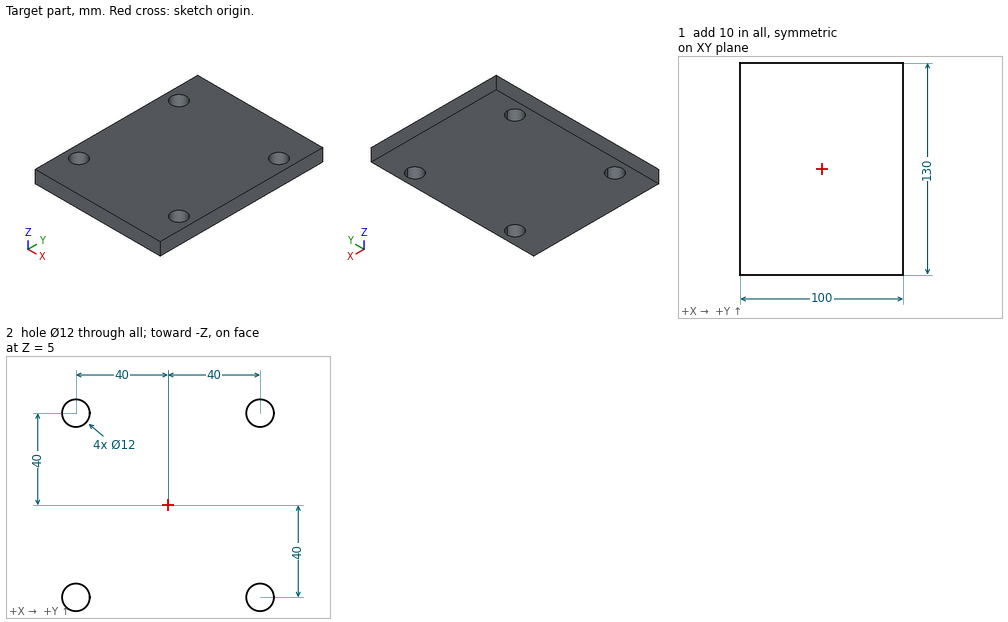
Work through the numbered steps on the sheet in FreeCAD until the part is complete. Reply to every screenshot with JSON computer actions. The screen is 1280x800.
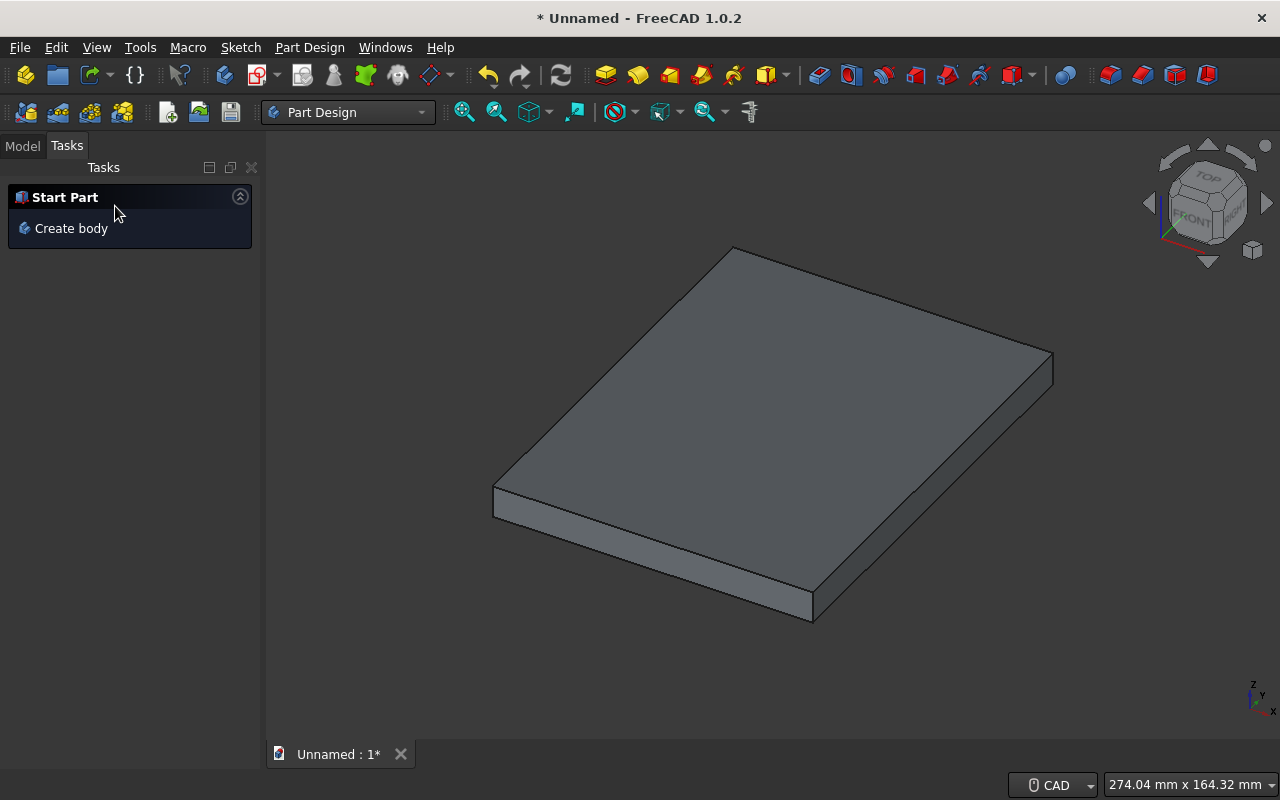
{"action": "left_click", "coordinate": [773, 419]}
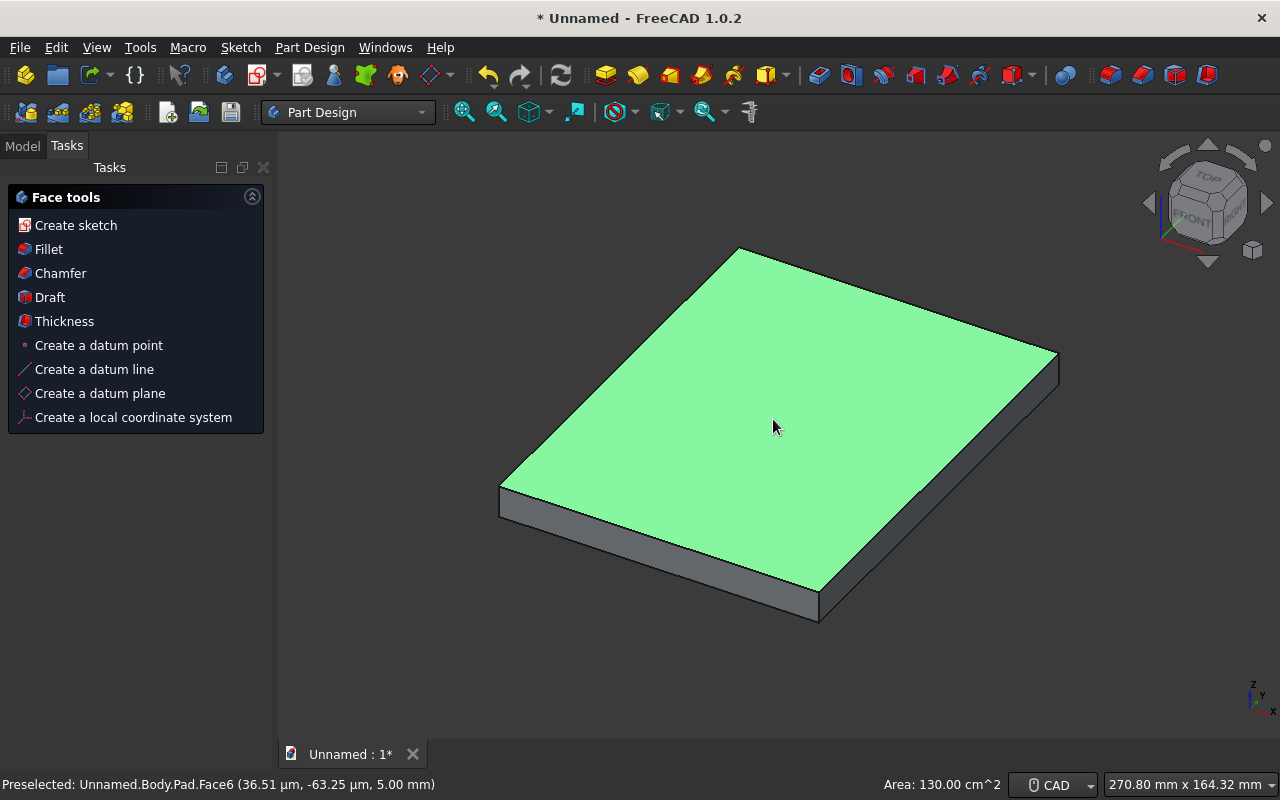
{"action": "left_click", "coordinate": [258, 76]}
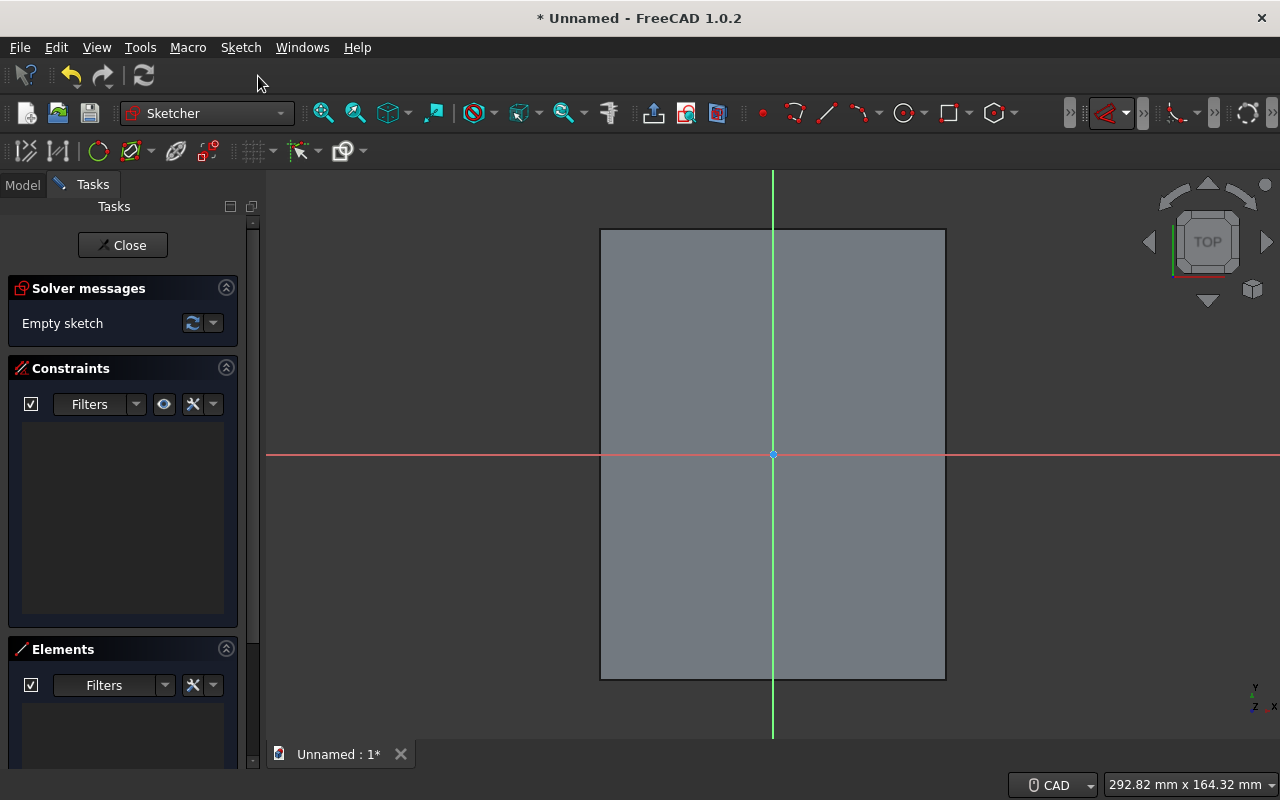
{"action": "left_click", "coordinate": [904, 114]}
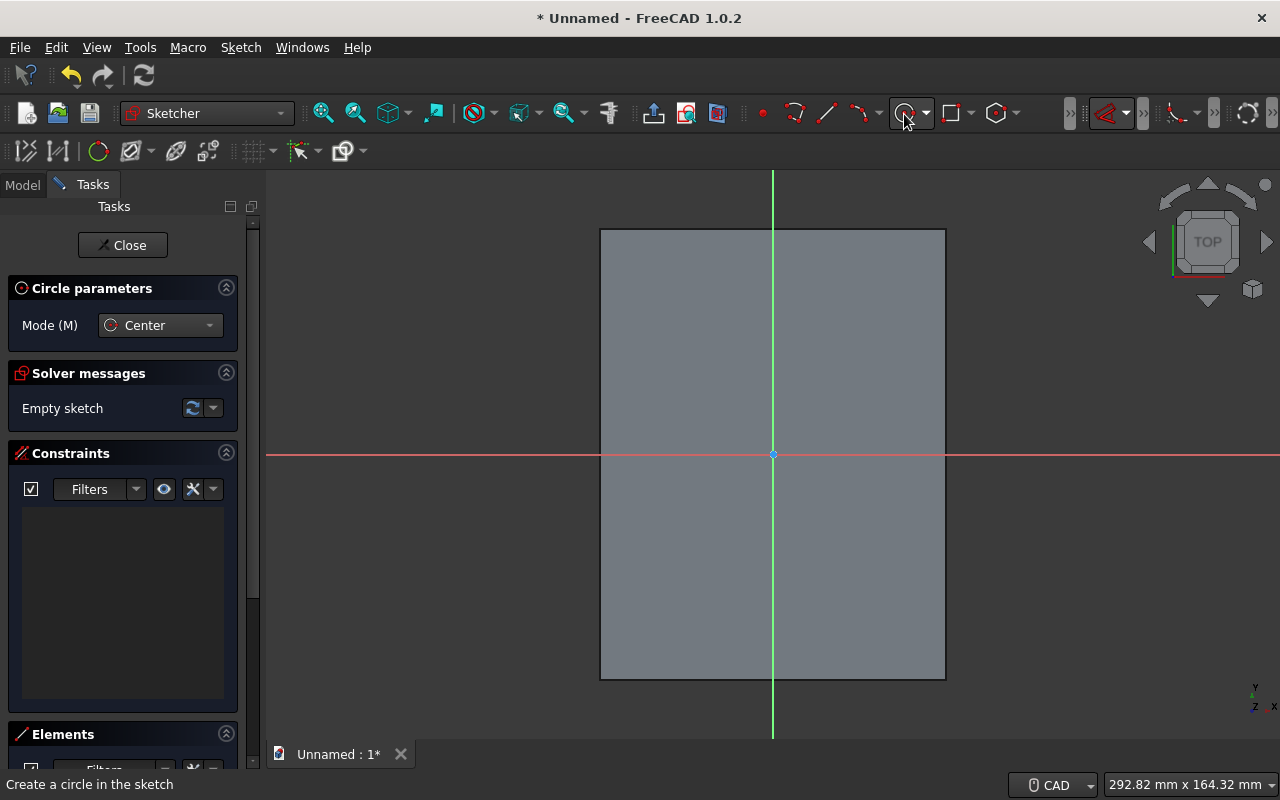
{"action": "left_click", "coordinate": [634, 316]}
{"action": "left_click", "coordinate": [649, 301]}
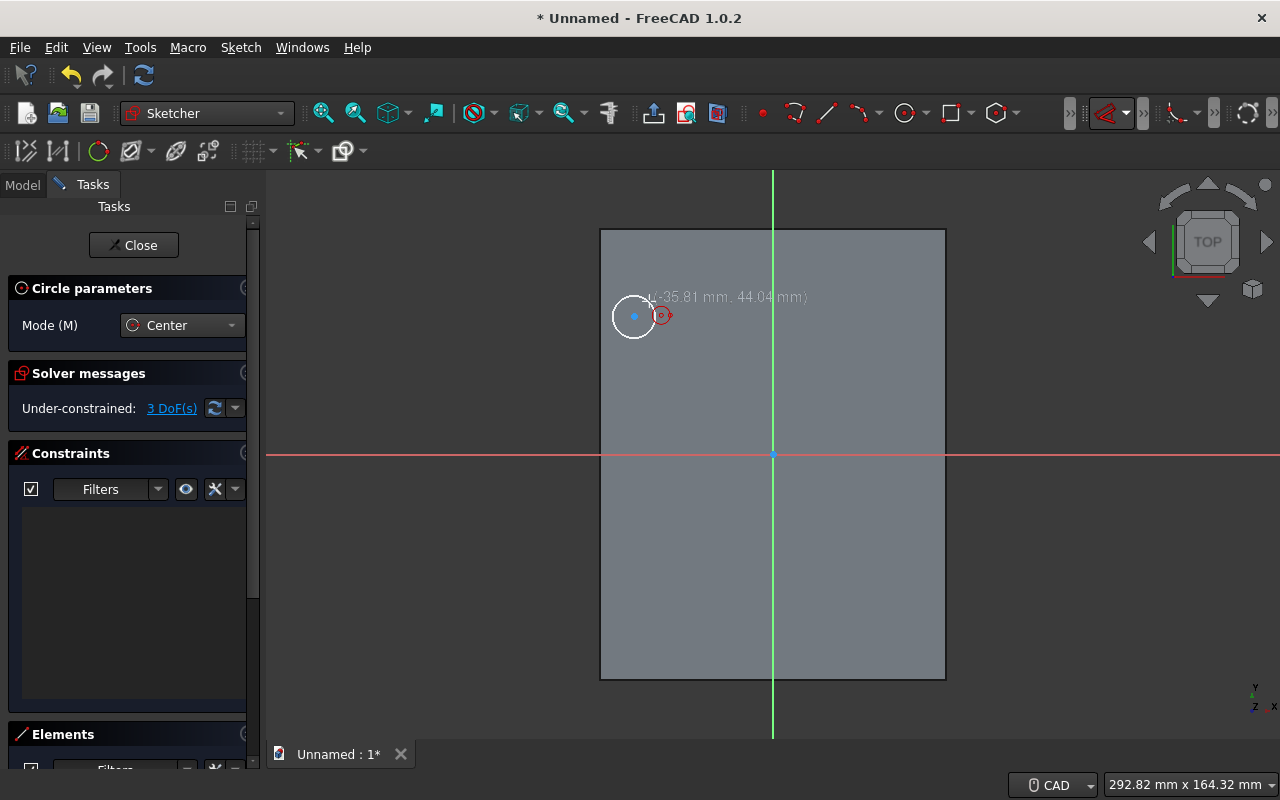
{"action": "left_click", "coordinate": [912, 316]}
{"action": "left_click", "coordinate": [926, 301]}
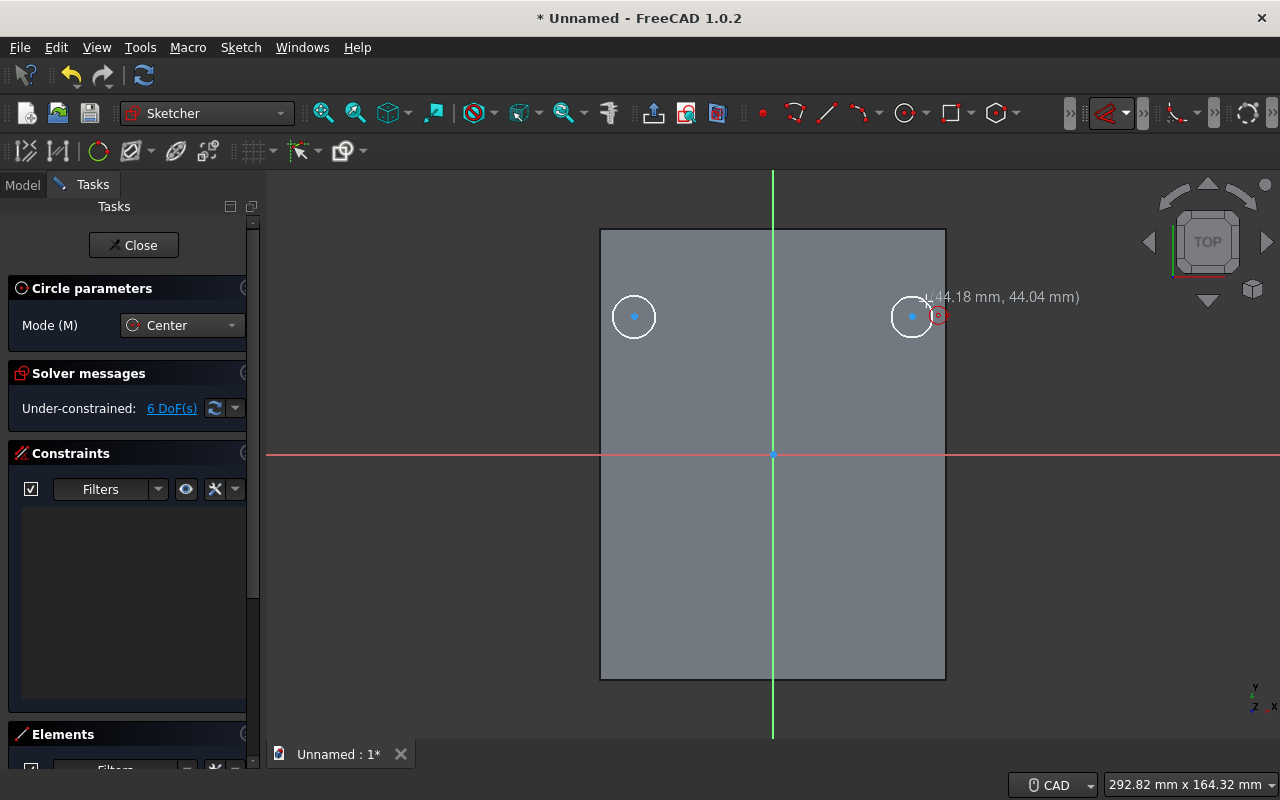
{"action": "left_click", "coordinate": [912, 593]}
{"action": "left_click", "coordinate": [926, 578]}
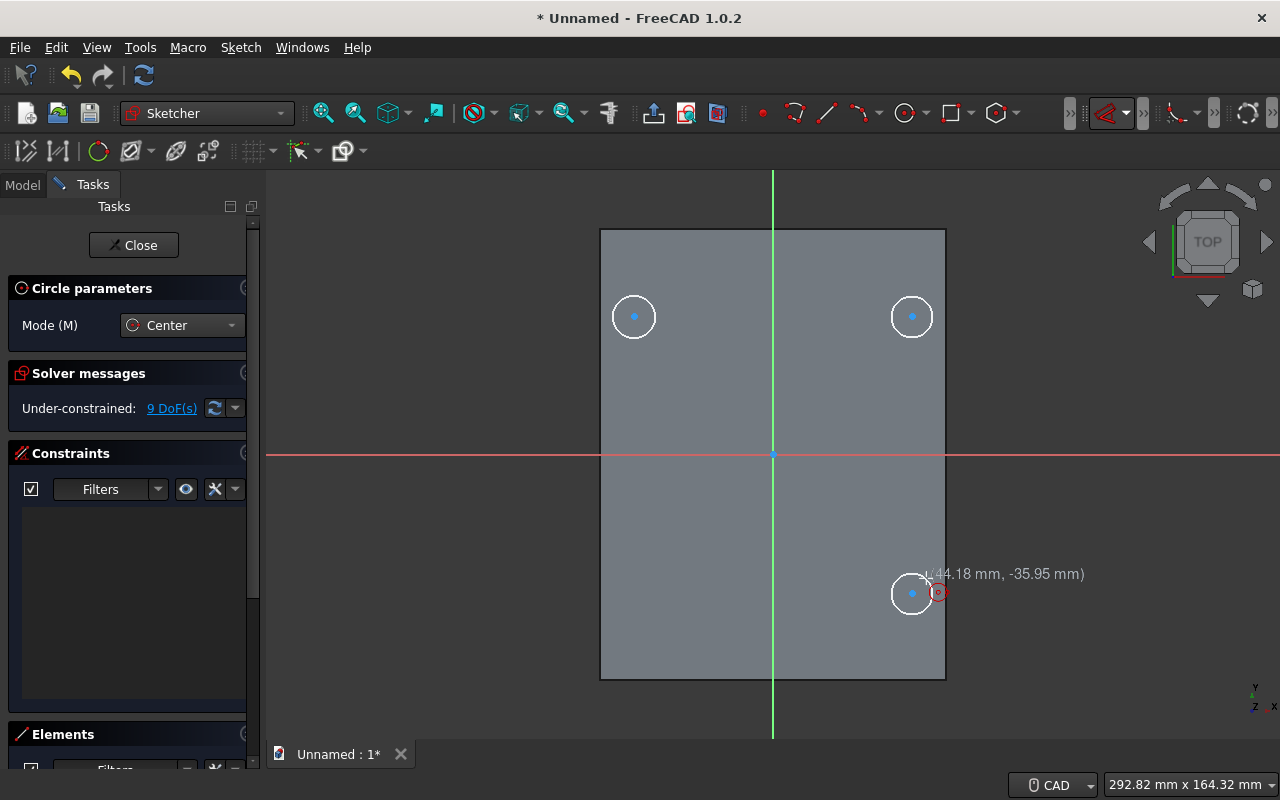
{"action": "left_click", "coordinate": [634, 593]}
{"action": "left_click", "coordinate": [649, 578]}
{"action": "key", "text": "Escape"}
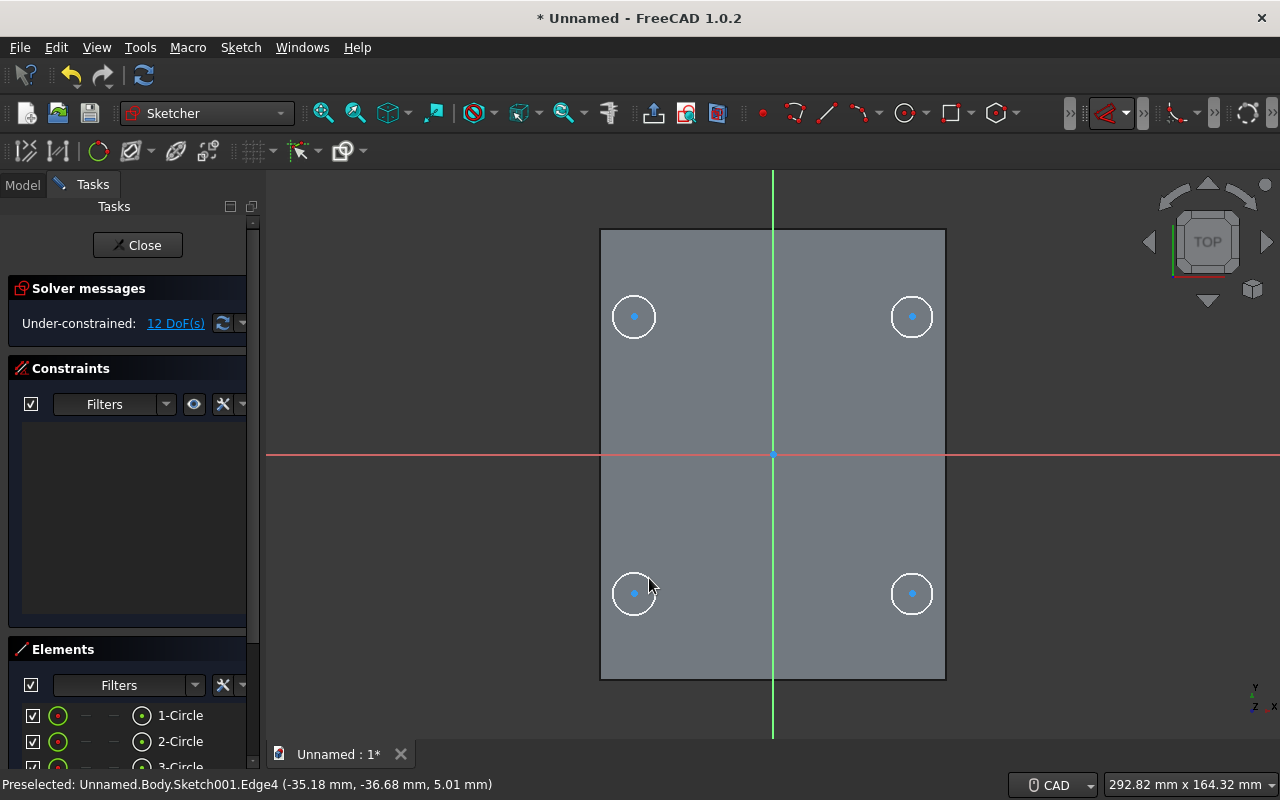
{"action": "left_click", "coordinate": [649, 302]}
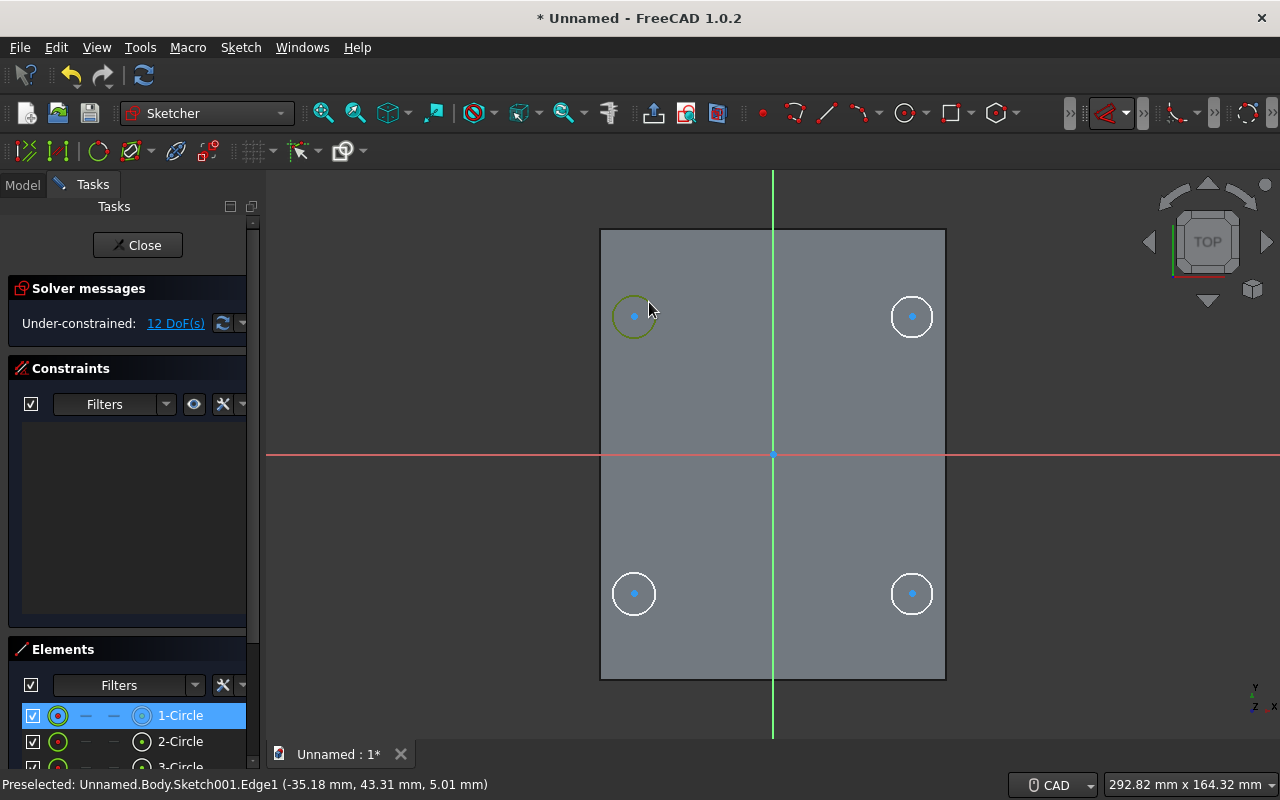
{"action": "left_click", "coordinate": [926, 302]}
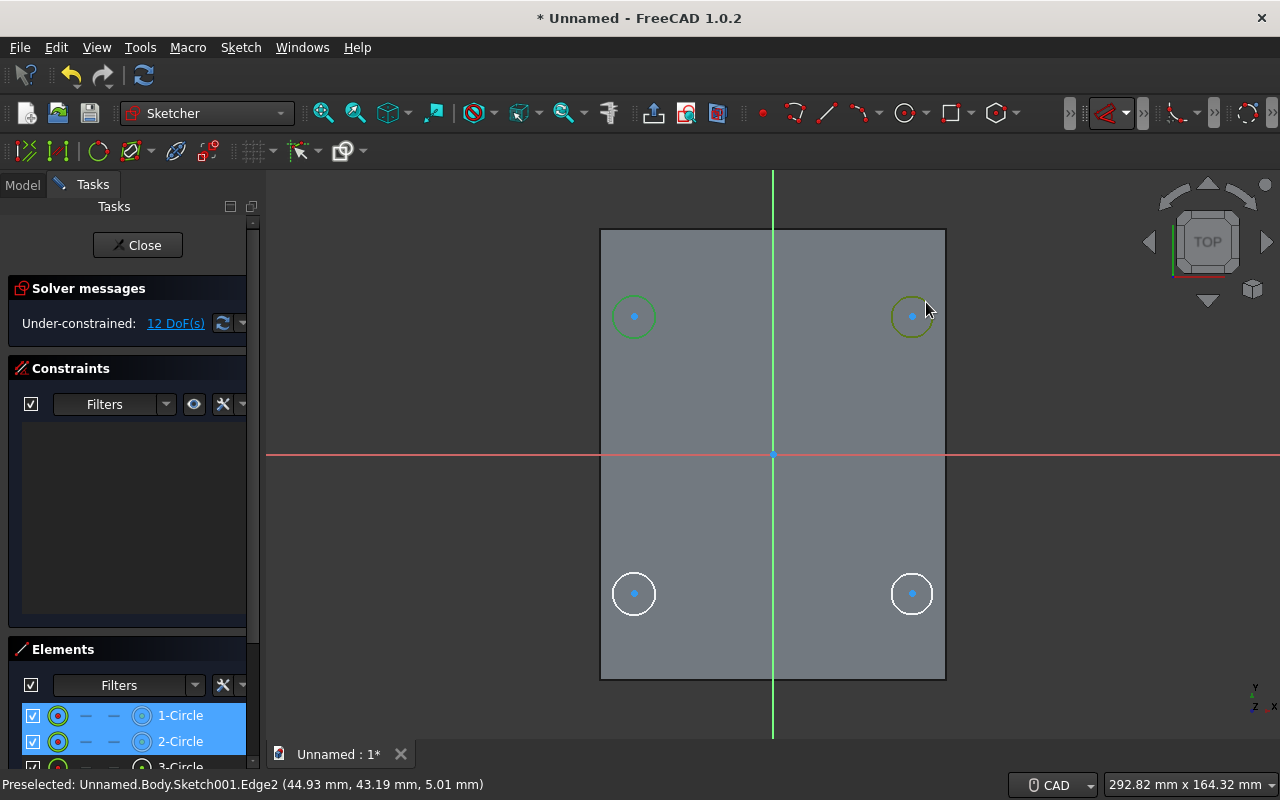
{"action": "left_click", "coordinate": [926, 579]}